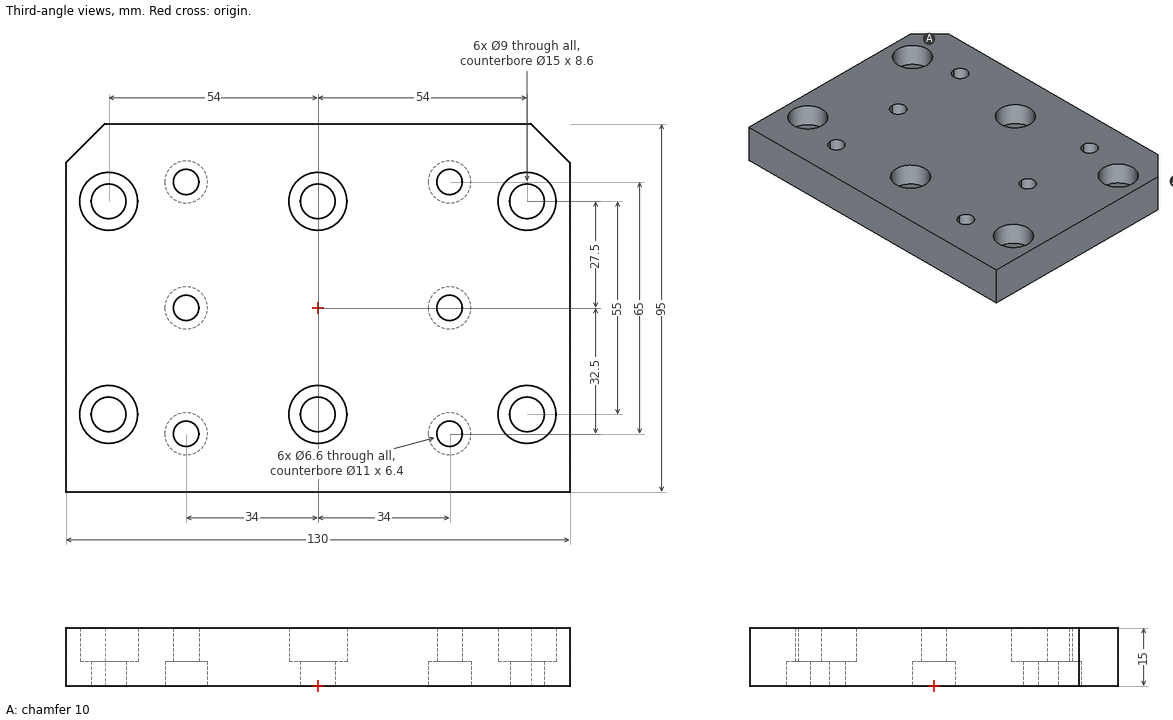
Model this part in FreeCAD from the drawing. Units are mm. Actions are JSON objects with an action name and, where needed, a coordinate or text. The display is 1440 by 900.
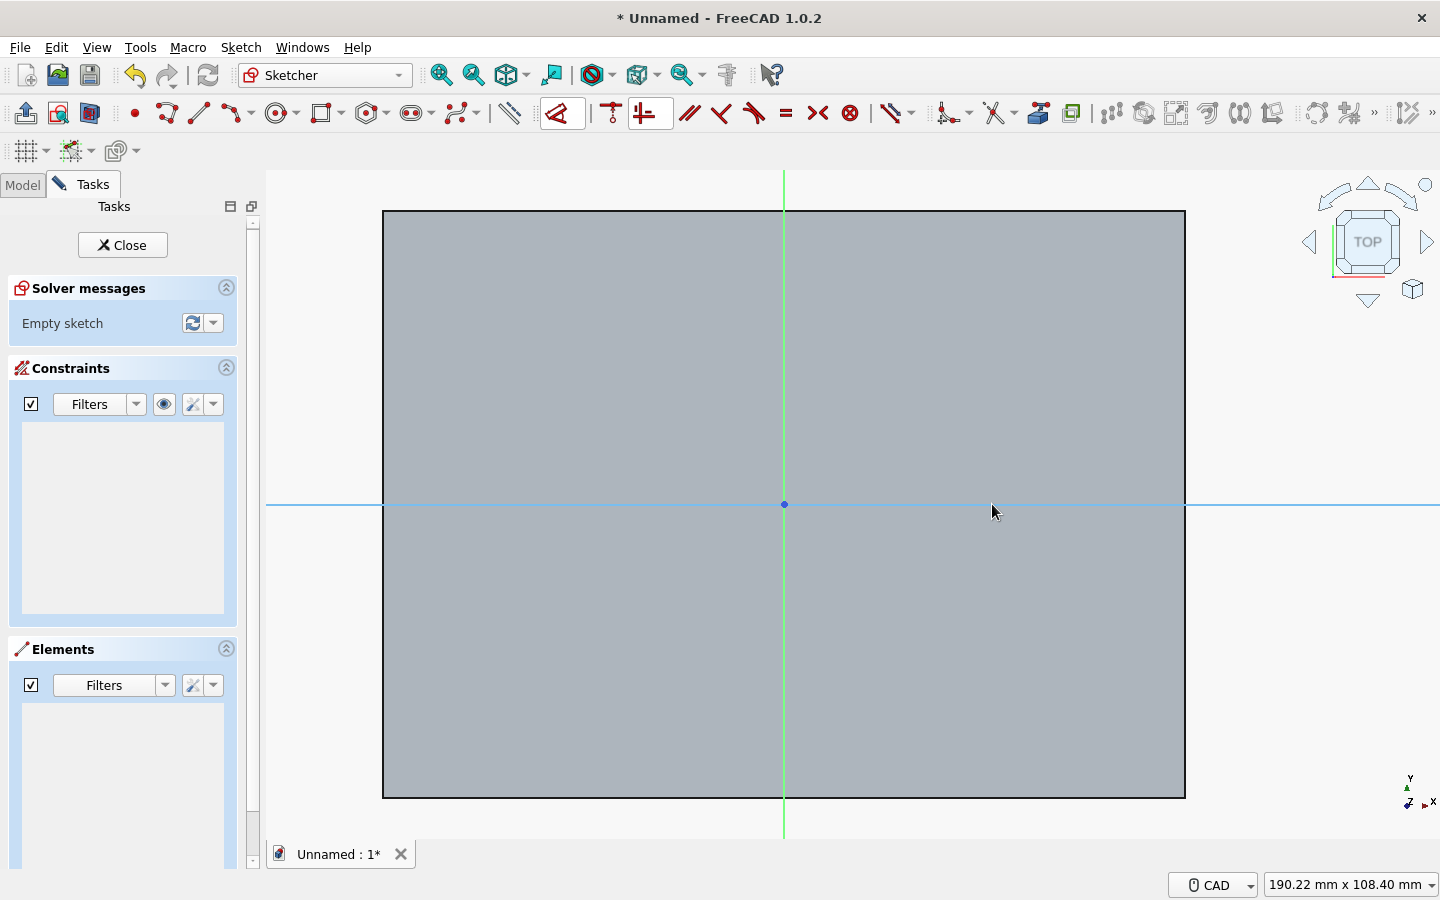
{"action": "left_click", "coordinate": [276, 114]}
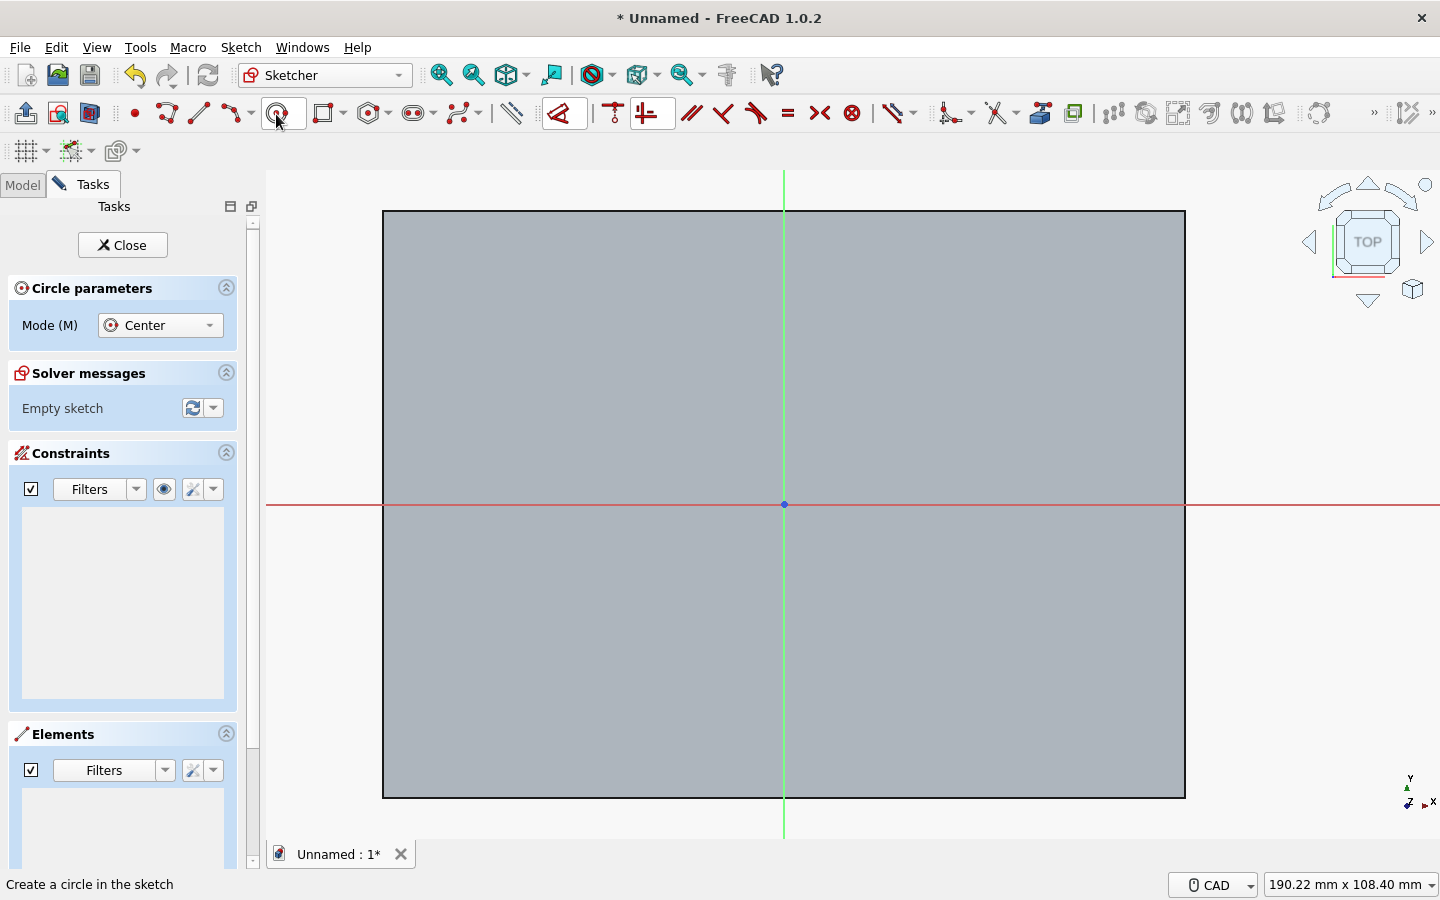
{"action": "left_click", "coordinate": [1118, 335]}
{"action": "mouse_move", "coordinate": [1137, 315]}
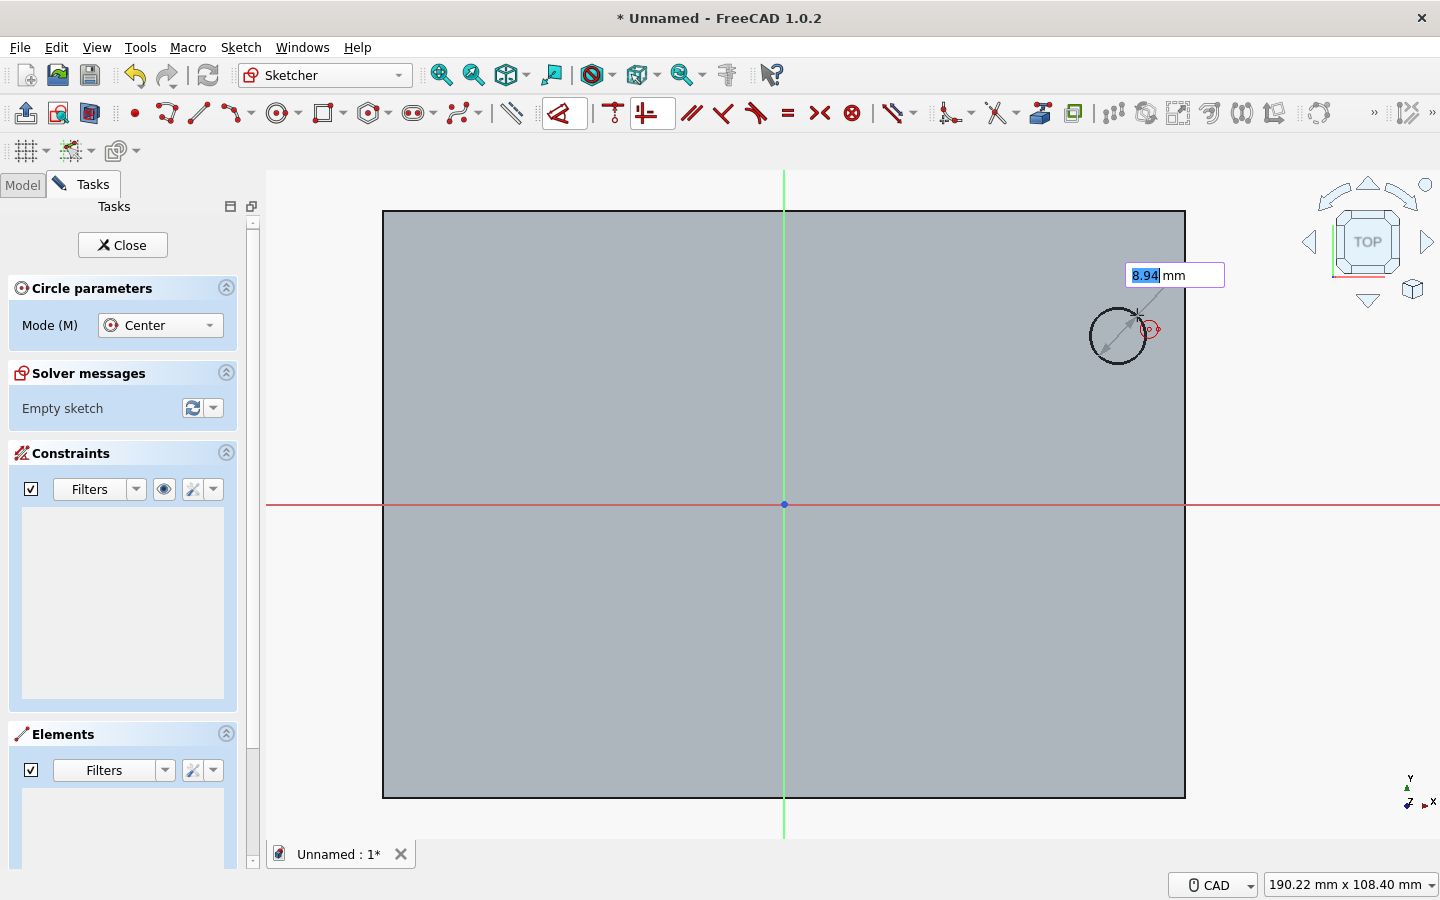
{"action": "type", "text": "9"}
{"action": "key", "text": "Return"}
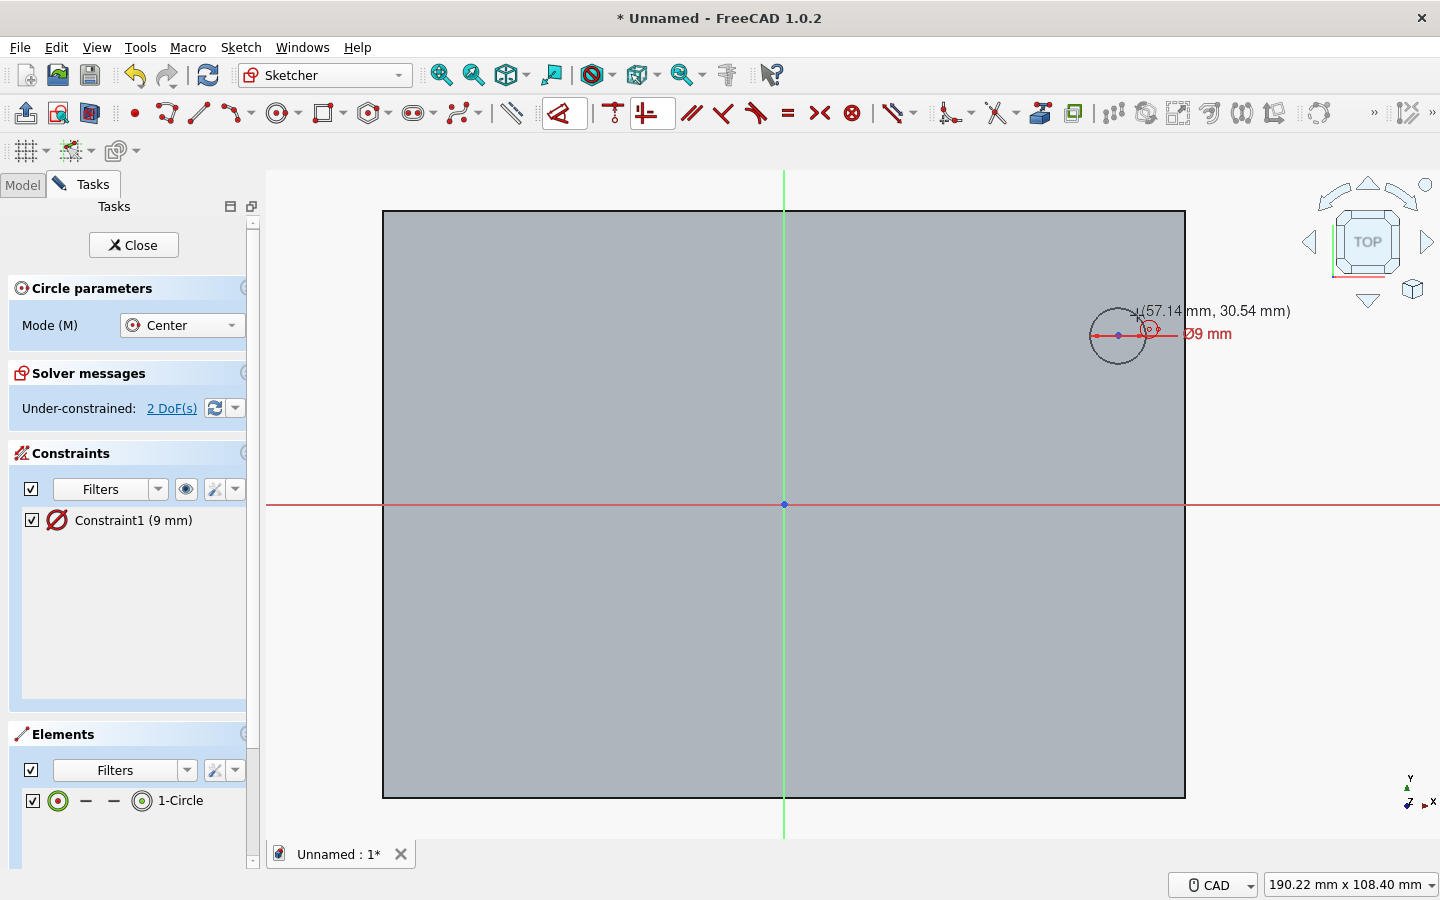
{"action": "left_click", "coordinate": [1118, 674]}
{"action": "mouse_move", "coordinate": [1137, 655]}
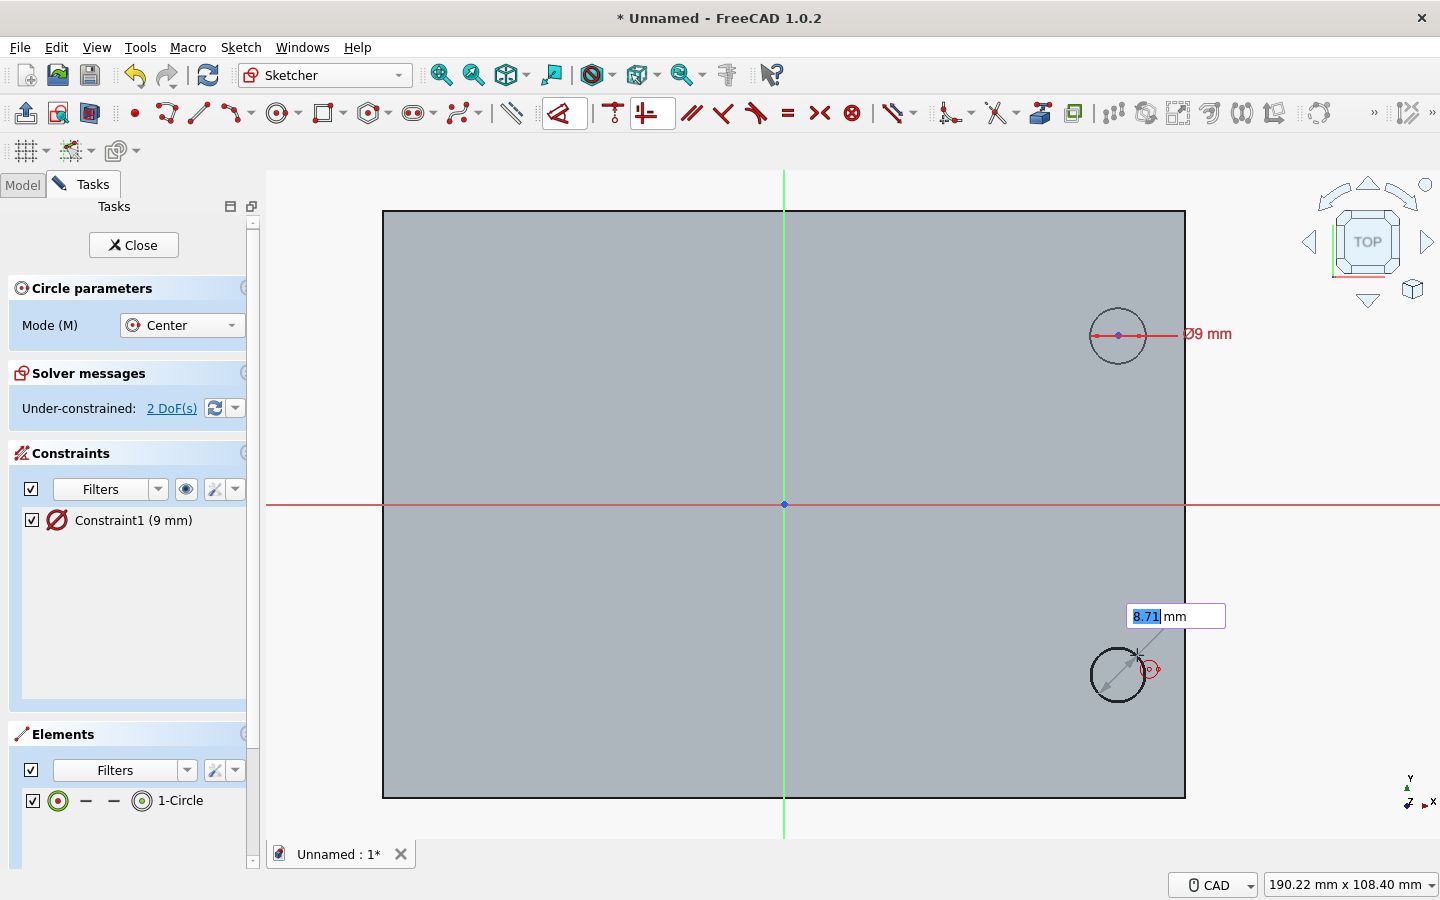
{"action": "type", "text": "9"}
{"action": "key", "text": "Return"}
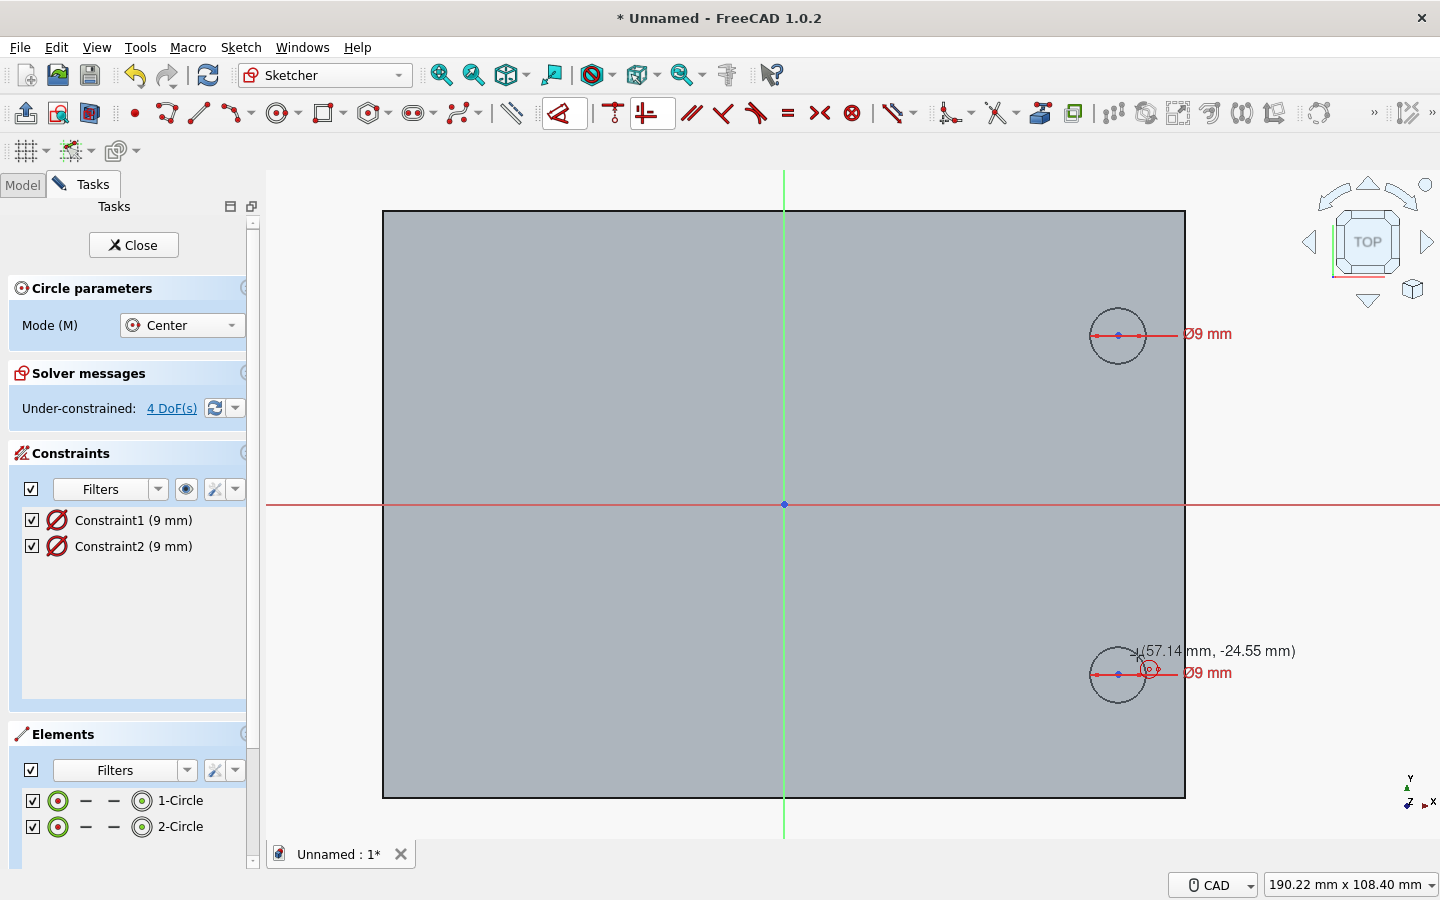
{"action": "left_click", "coordinate": [451, 335]}
{"action": "mouse_move", "coordinate": [471, 315]}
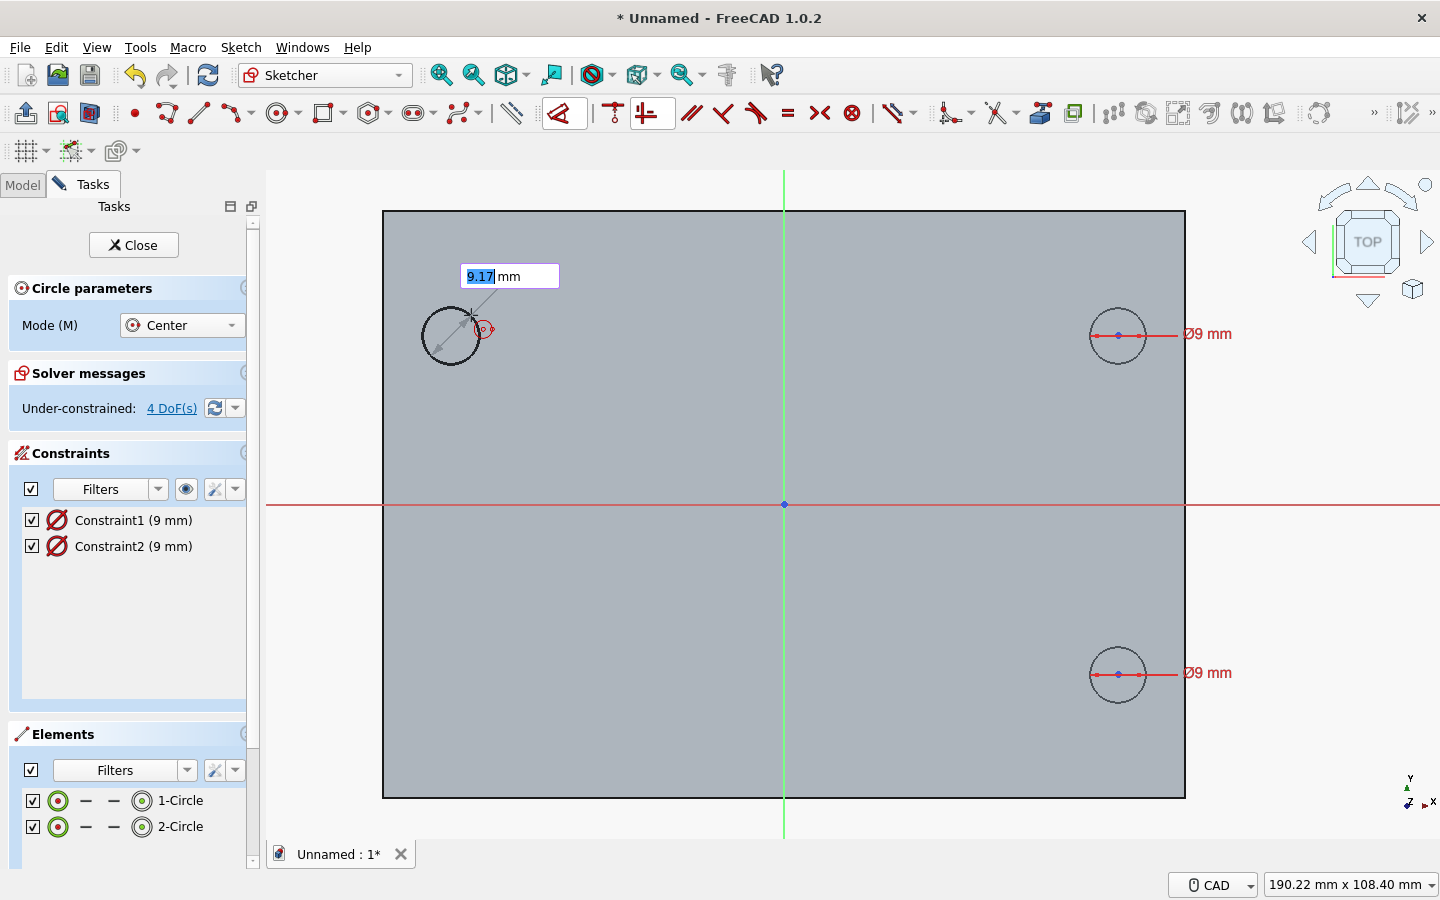
{"action": "type", "text": "9"}
{"action": "key", "text": "Return"}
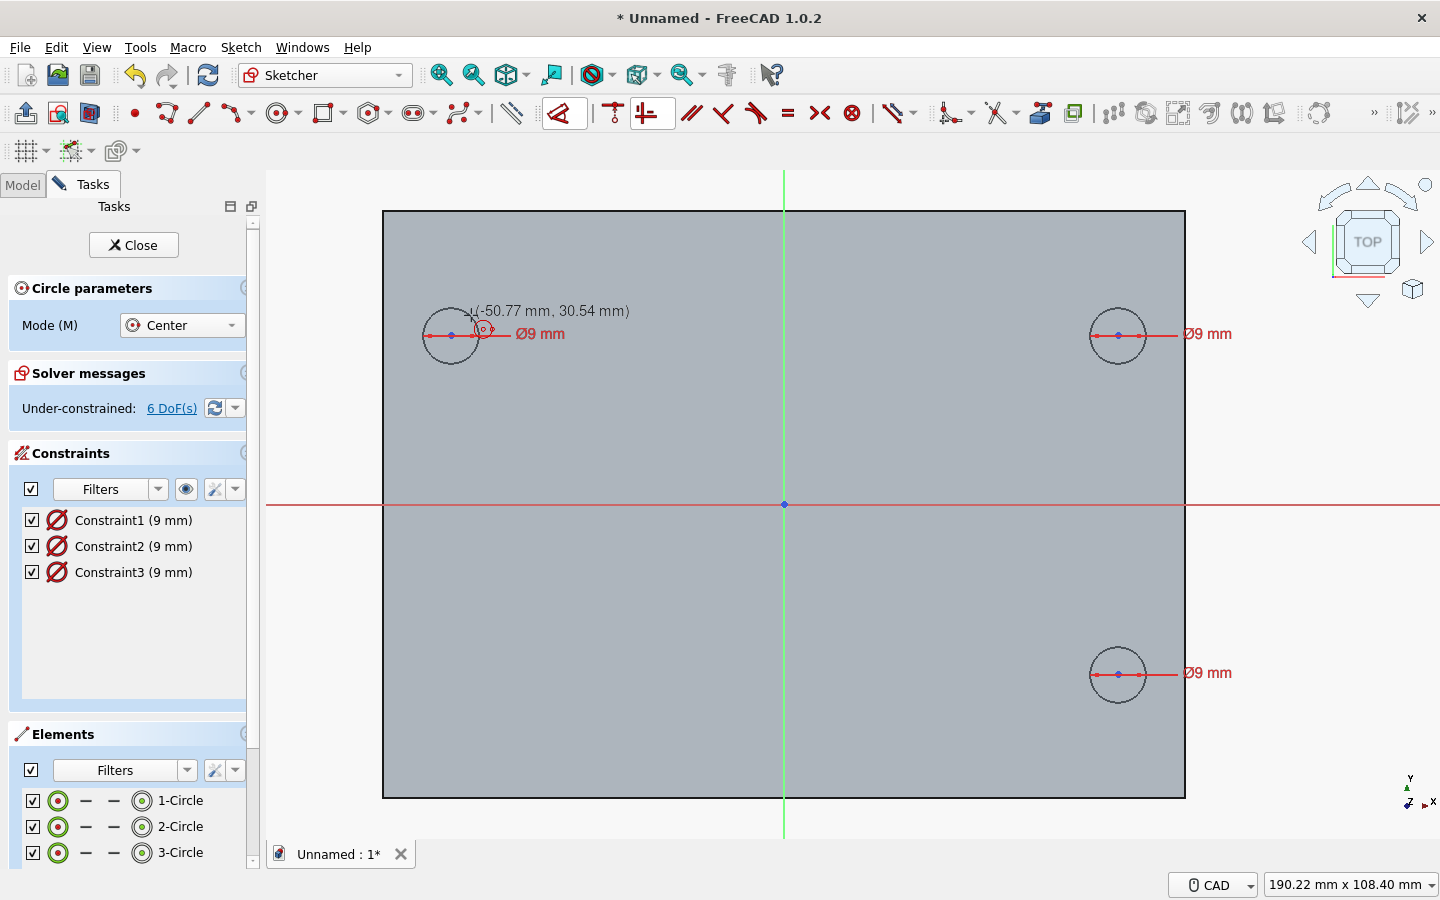
{"action": "left_click", "coordinate": [451, 674]}
{"action": "mouse_move", "coordinate": [471, 655]}